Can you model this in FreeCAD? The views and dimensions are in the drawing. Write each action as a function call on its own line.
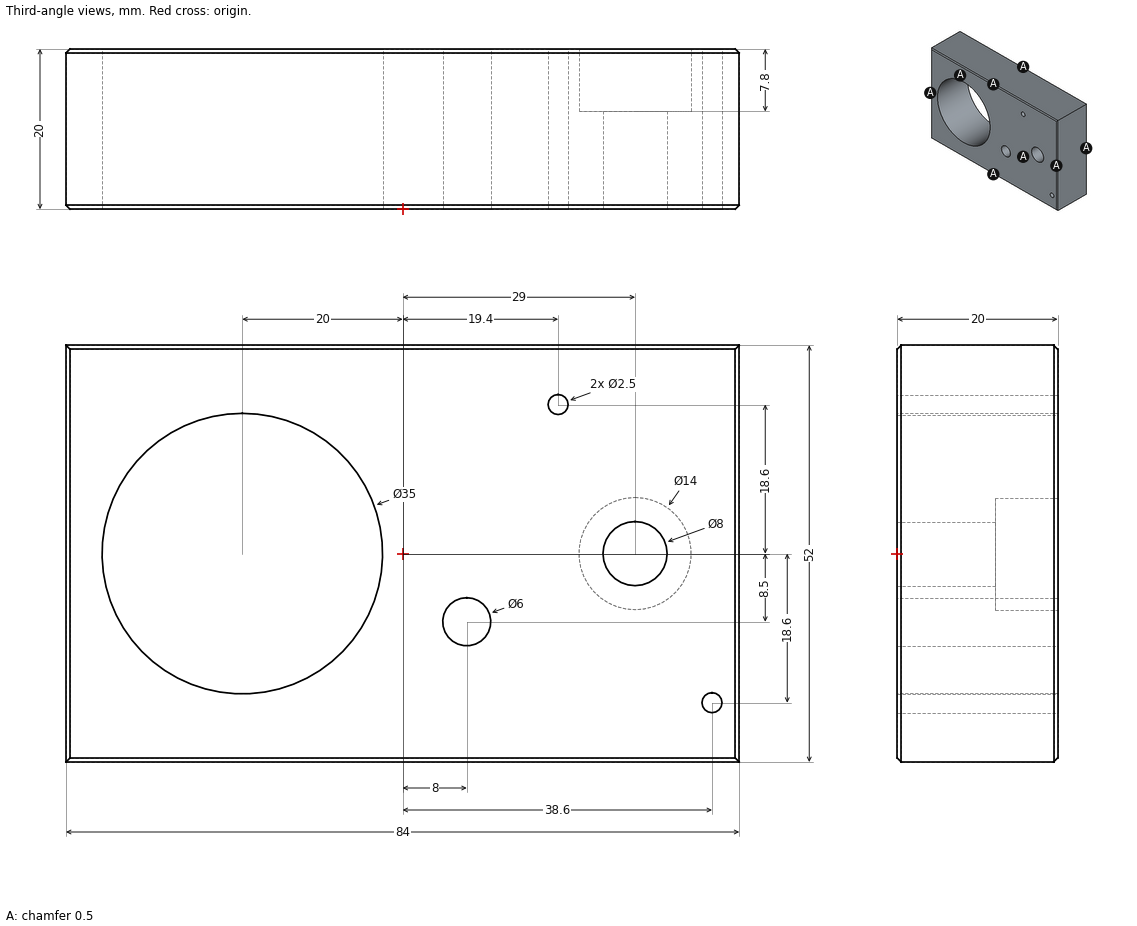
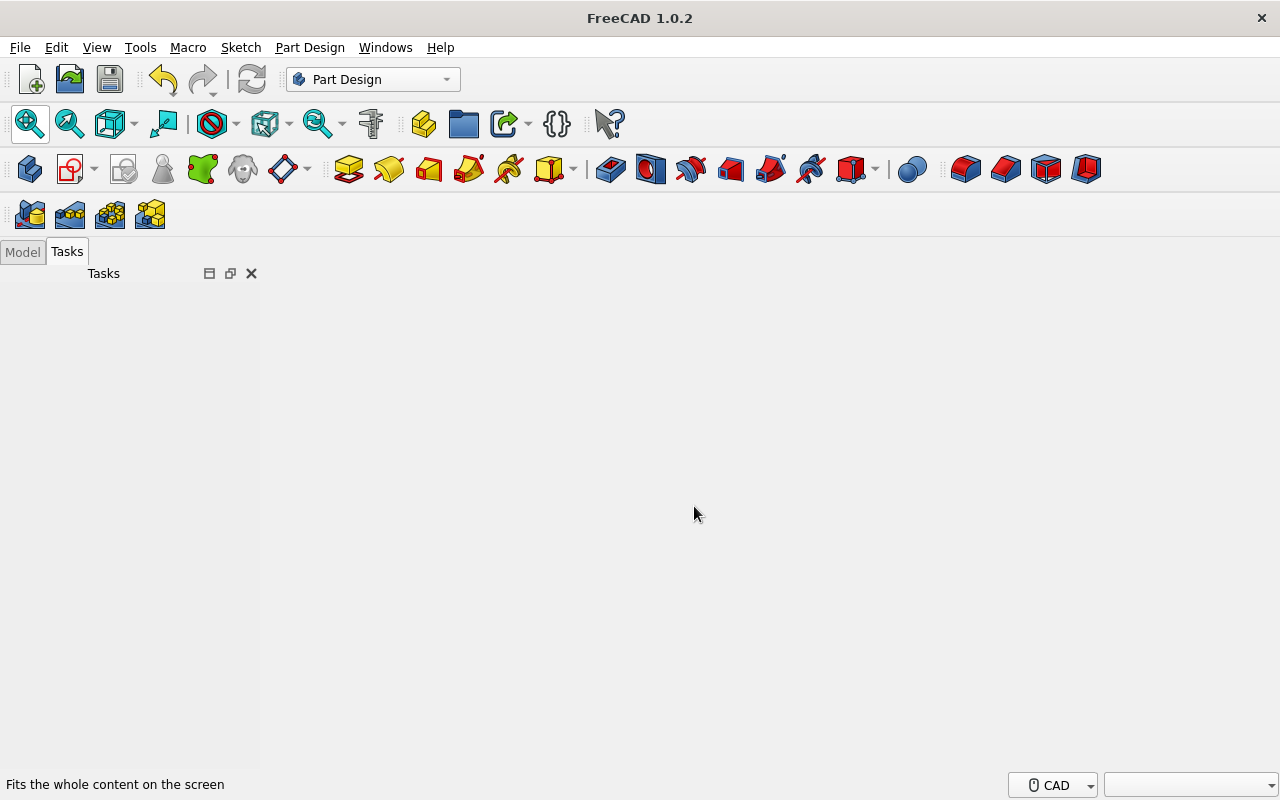
click(30, 80)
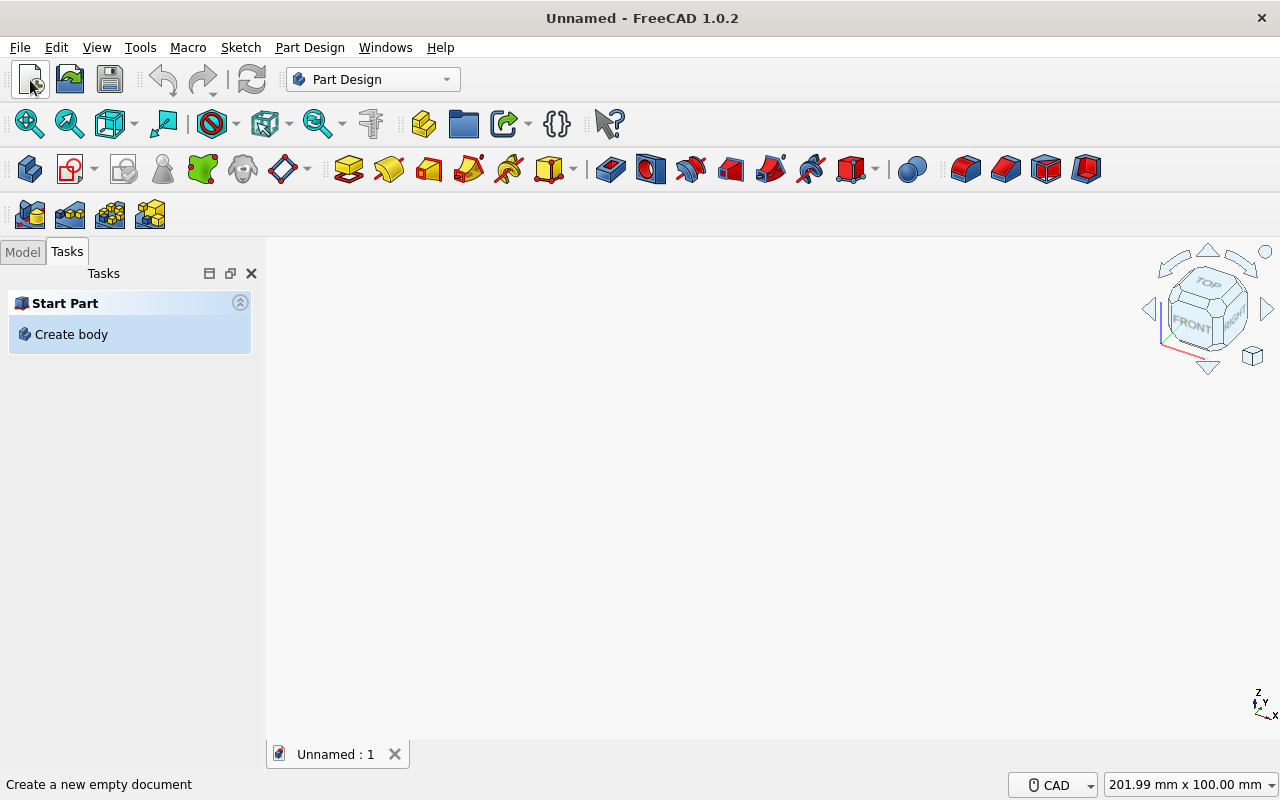
click(70, 170)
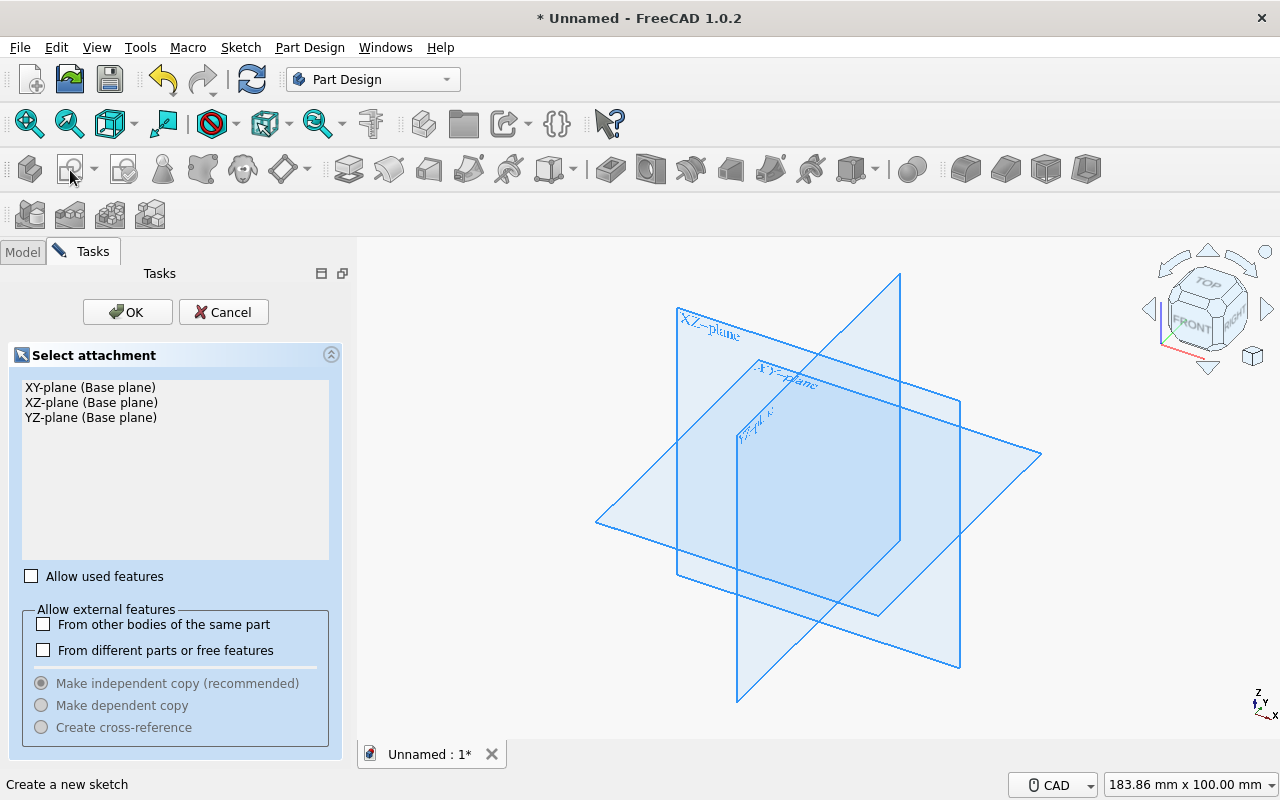
click(82, 402)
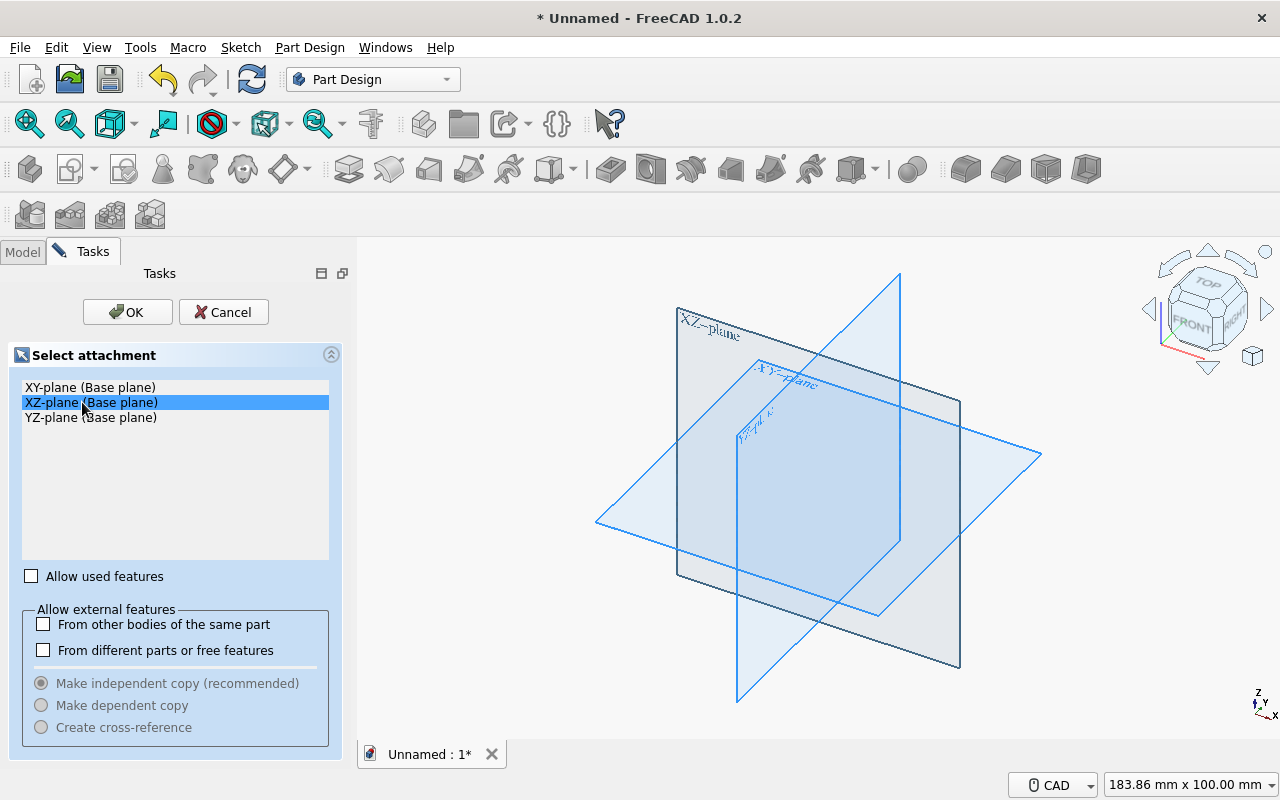
click(128, 312)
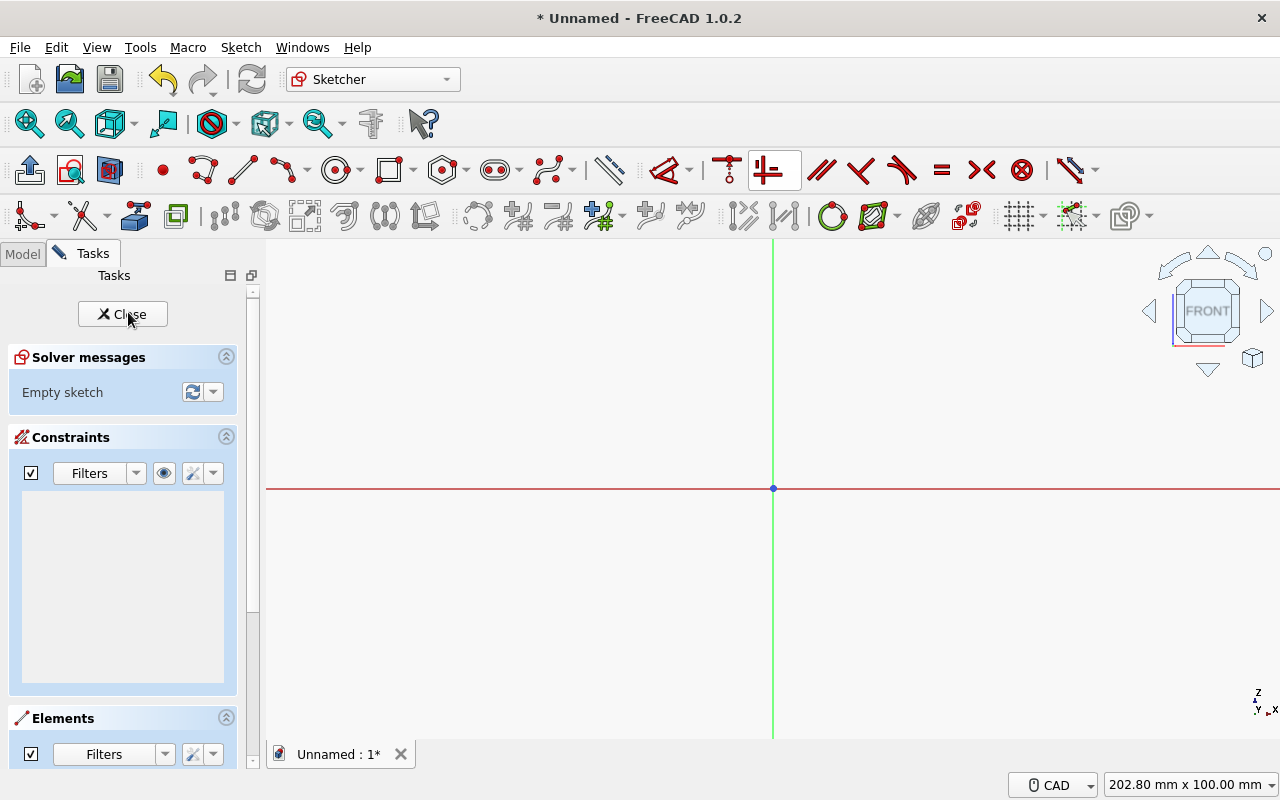
click(416, 170)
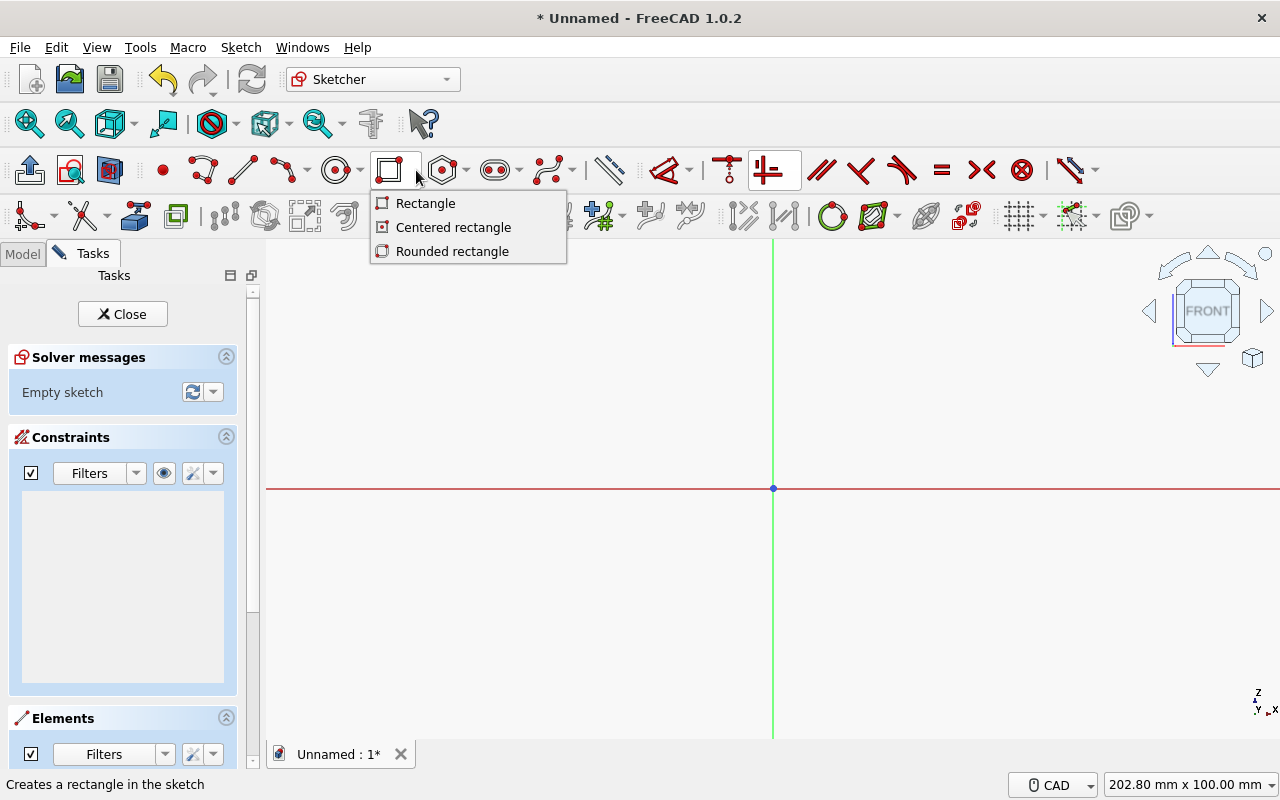
click(468, 227)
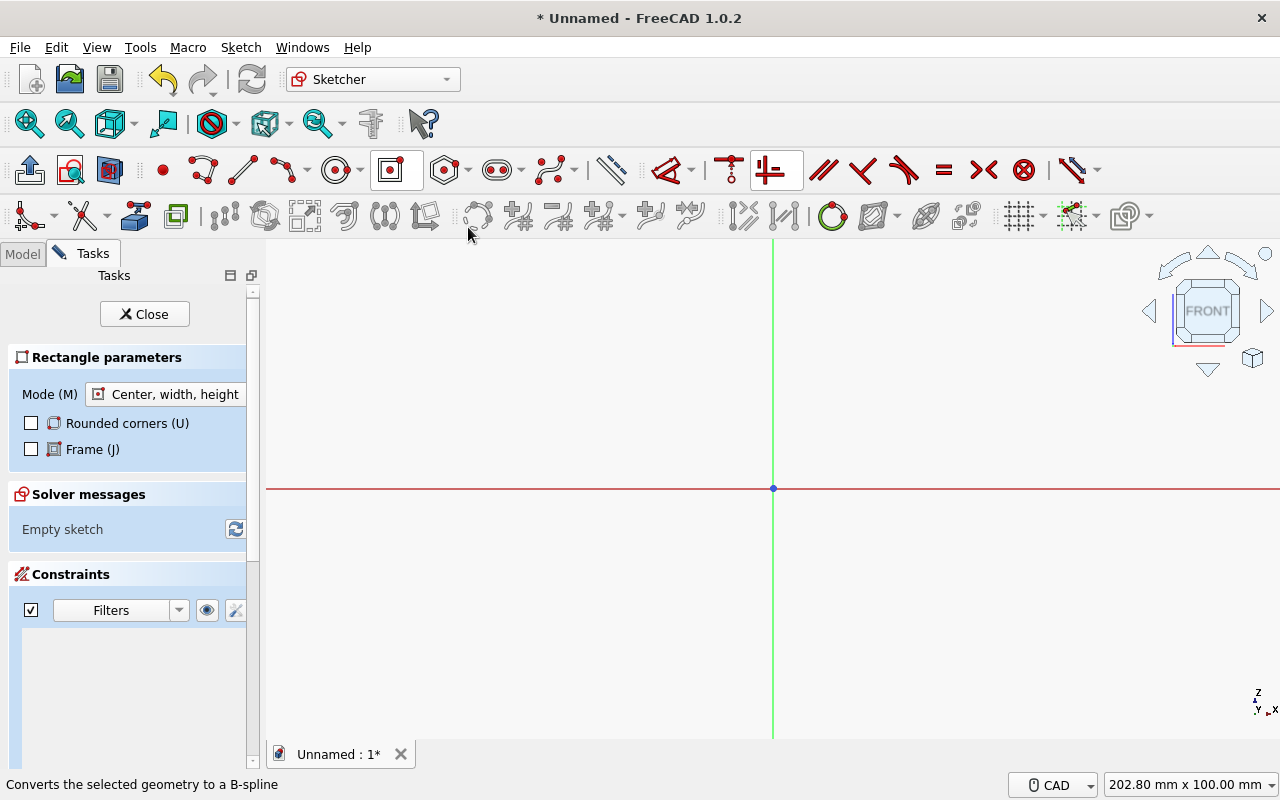
click(773, 489)
move(983, 359)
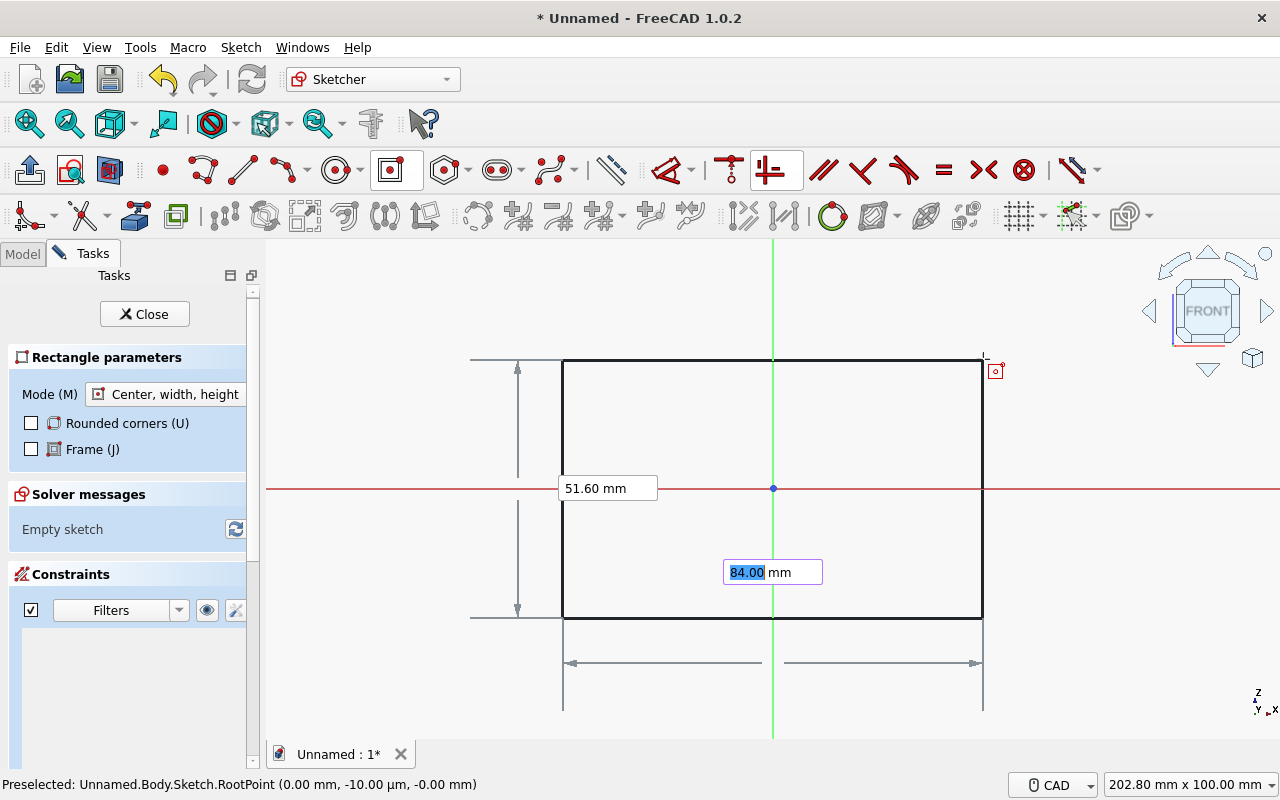
text(84)
key(Tab)
text(52)
key(Return)
key(Escape)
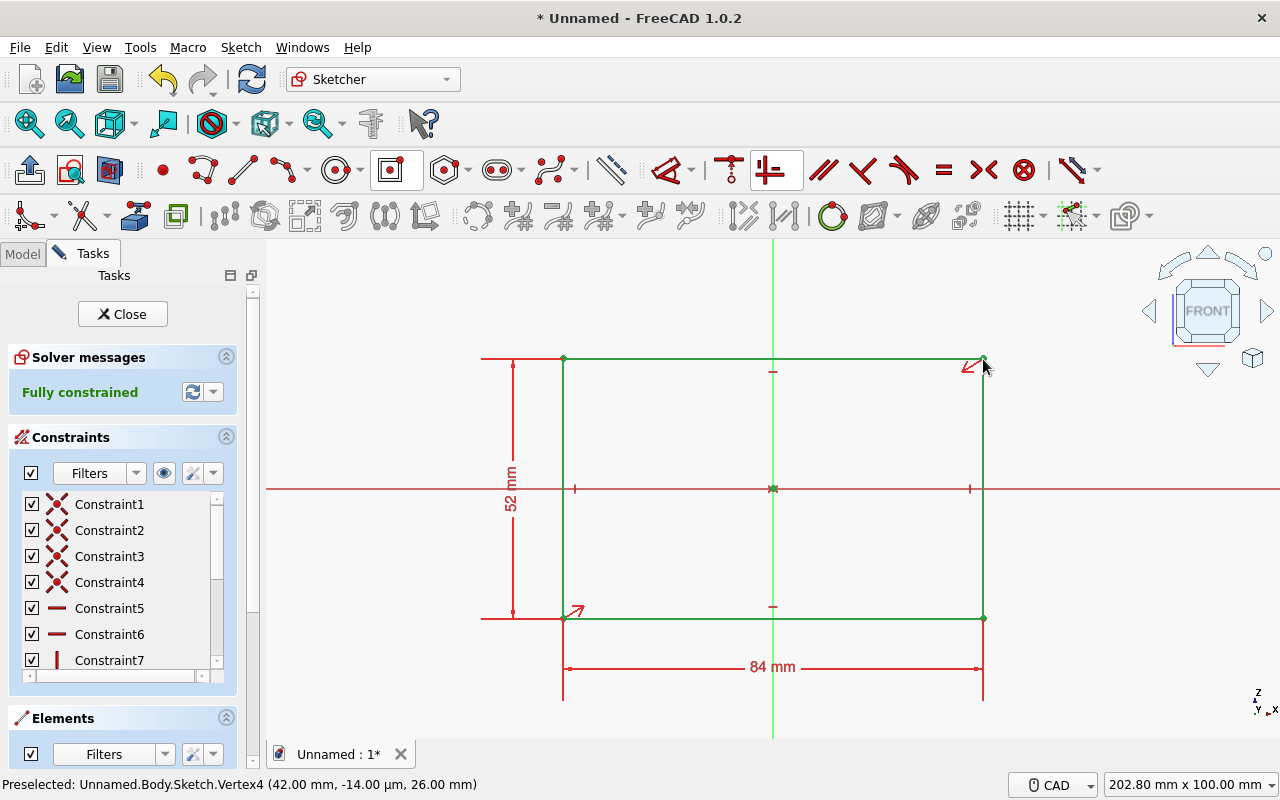
click(123, 314)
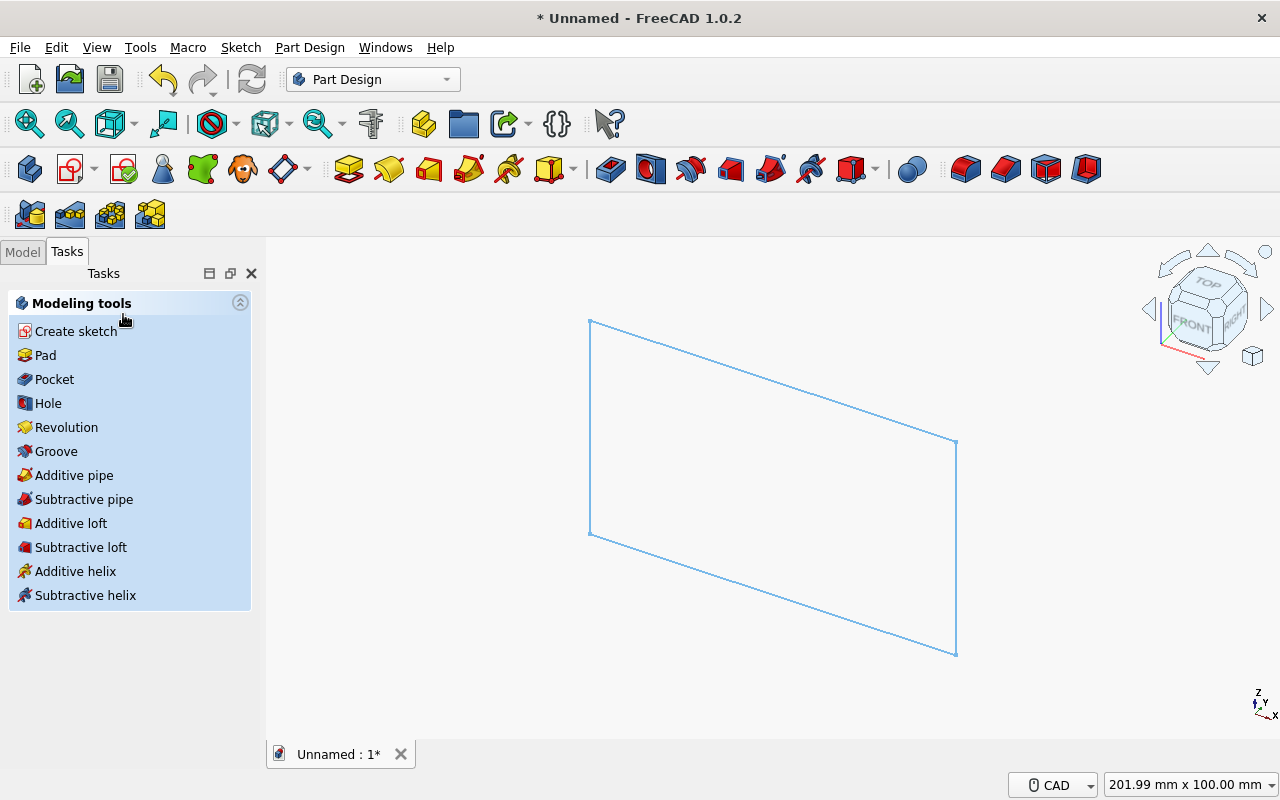
click(350, 170)